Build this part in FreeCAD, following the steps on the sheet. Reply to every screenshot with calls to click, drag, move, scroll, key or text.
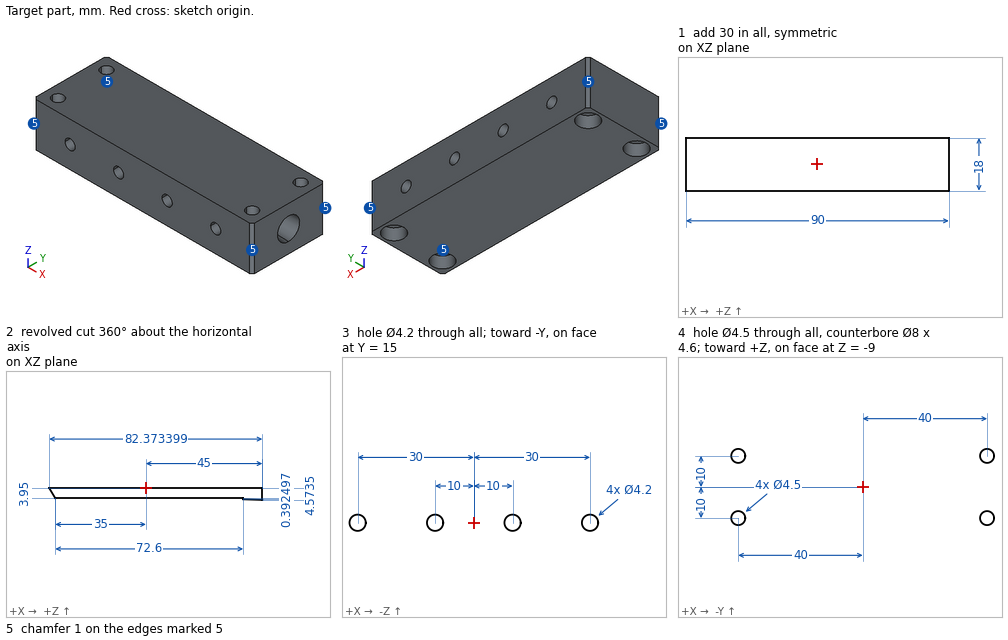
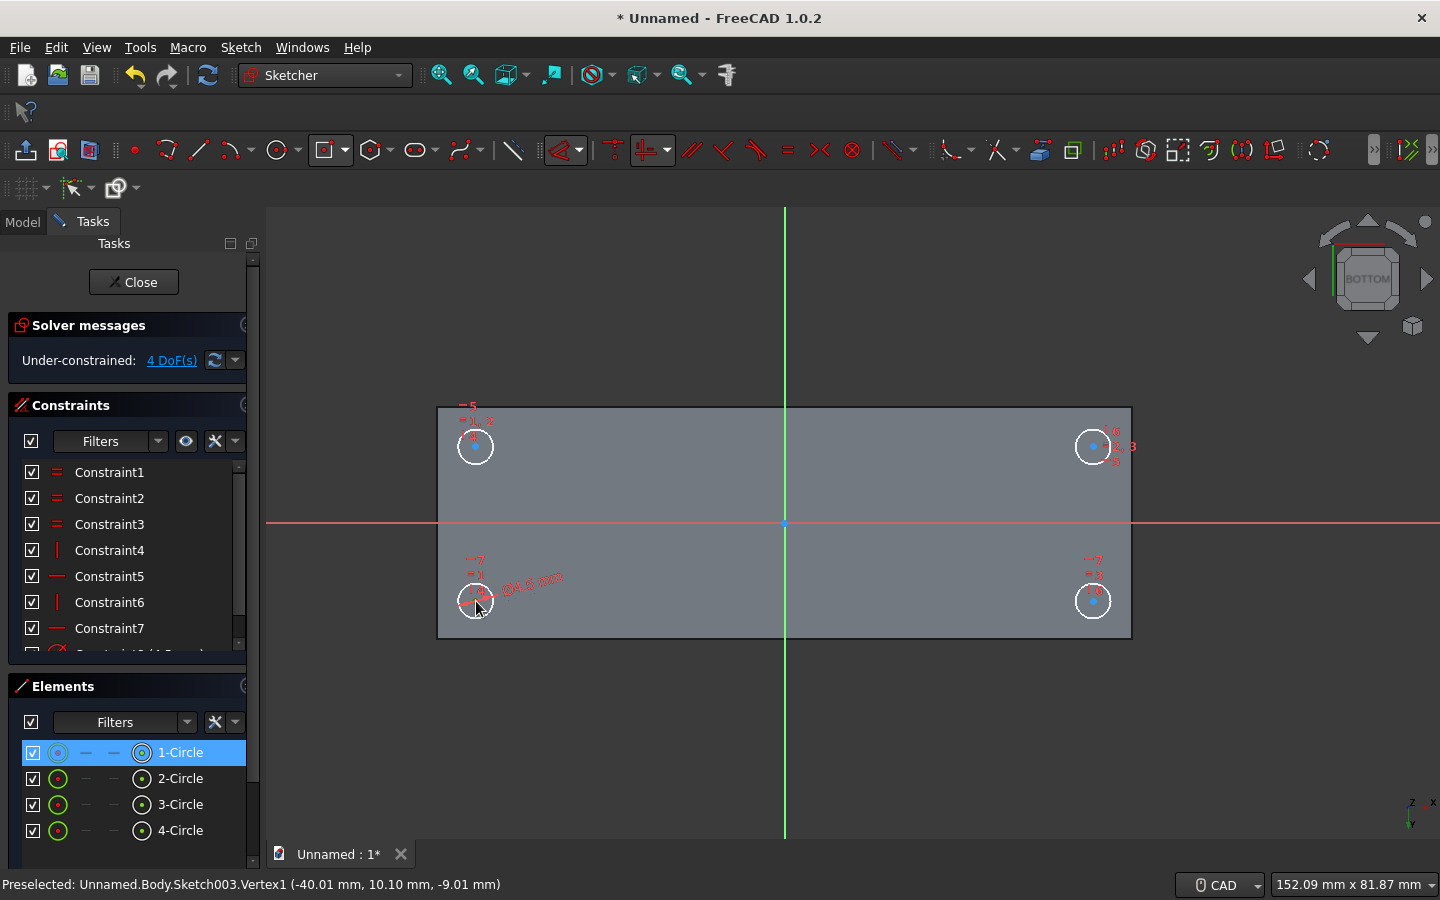
click(582, 150)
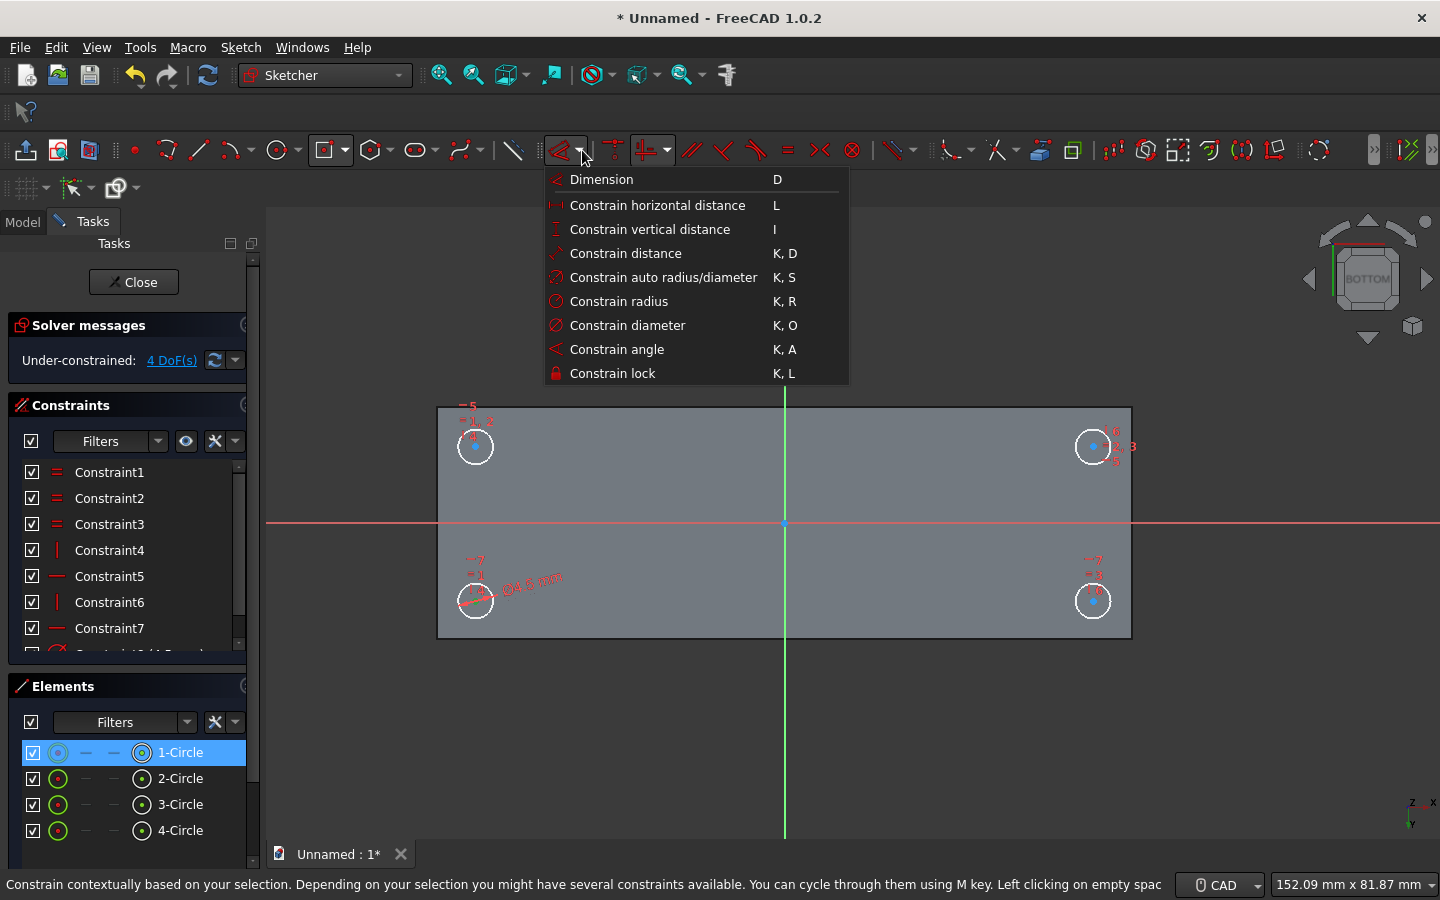
click(697, 205)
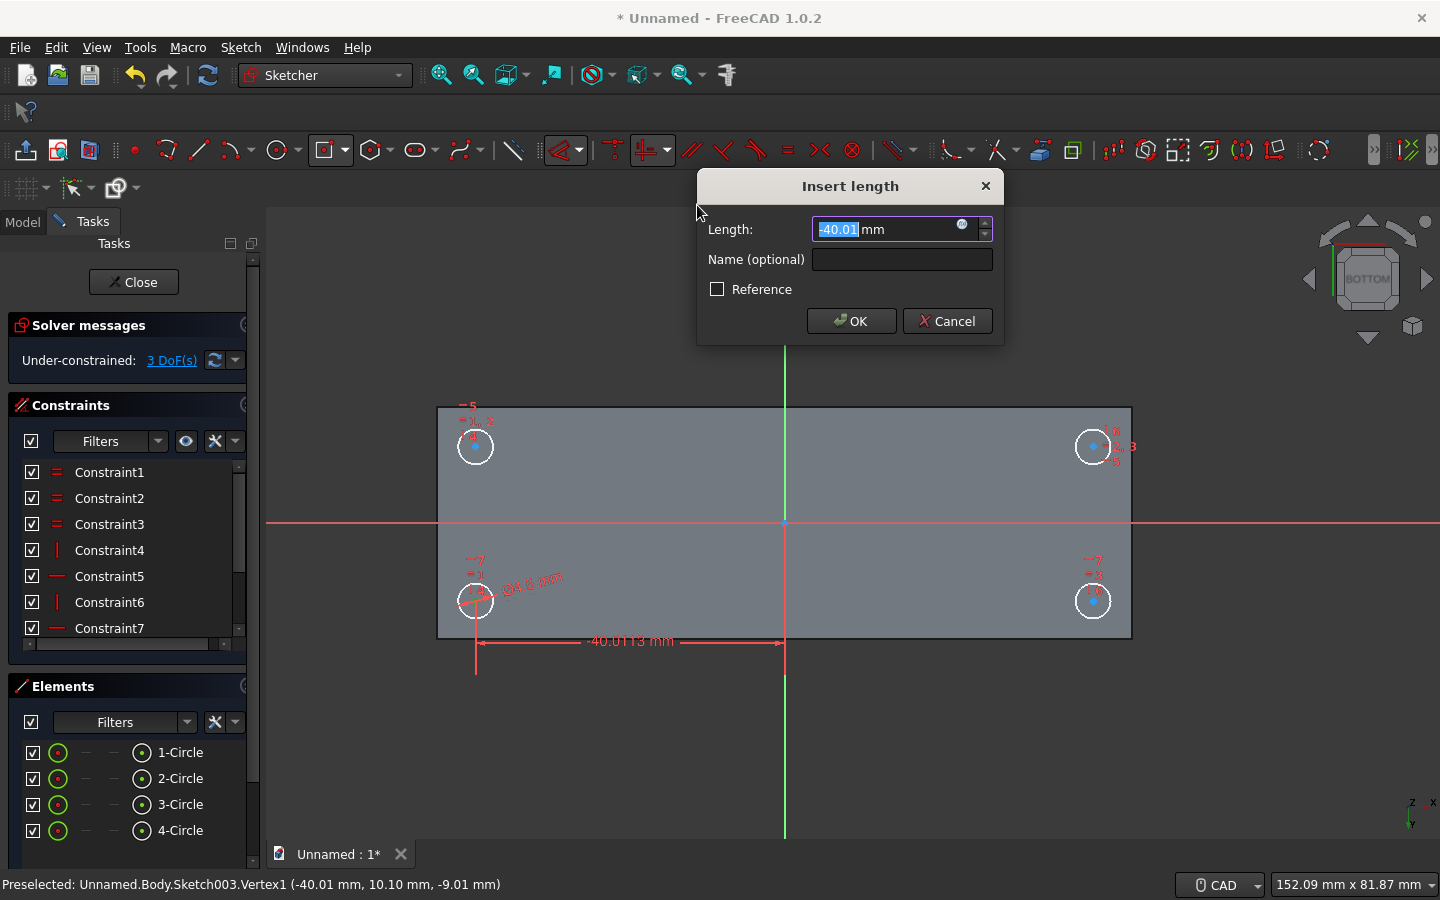
text(-40)
key(Return)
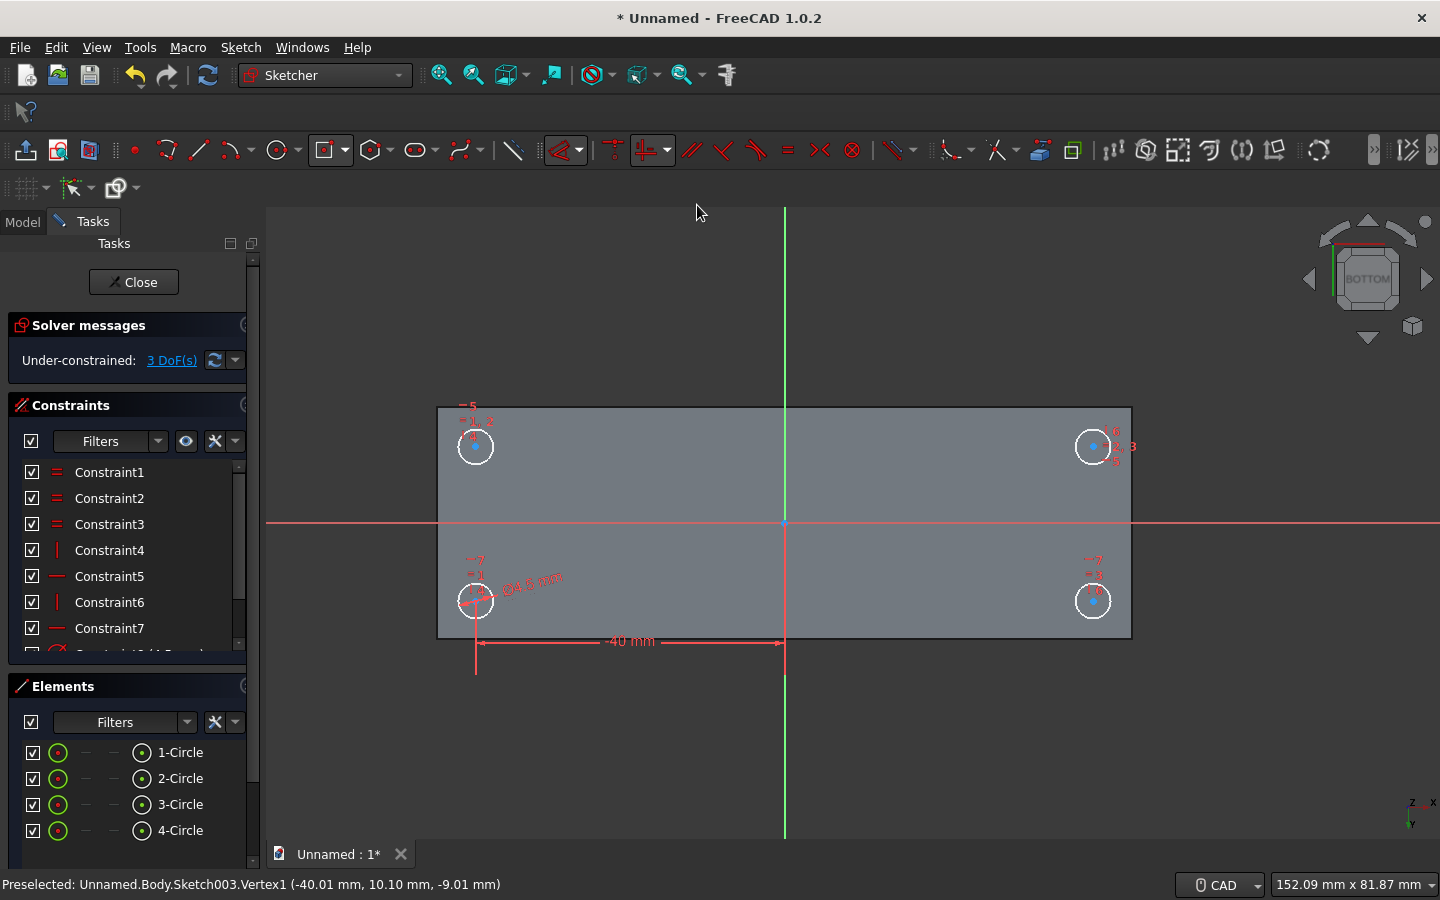
click(476, 601)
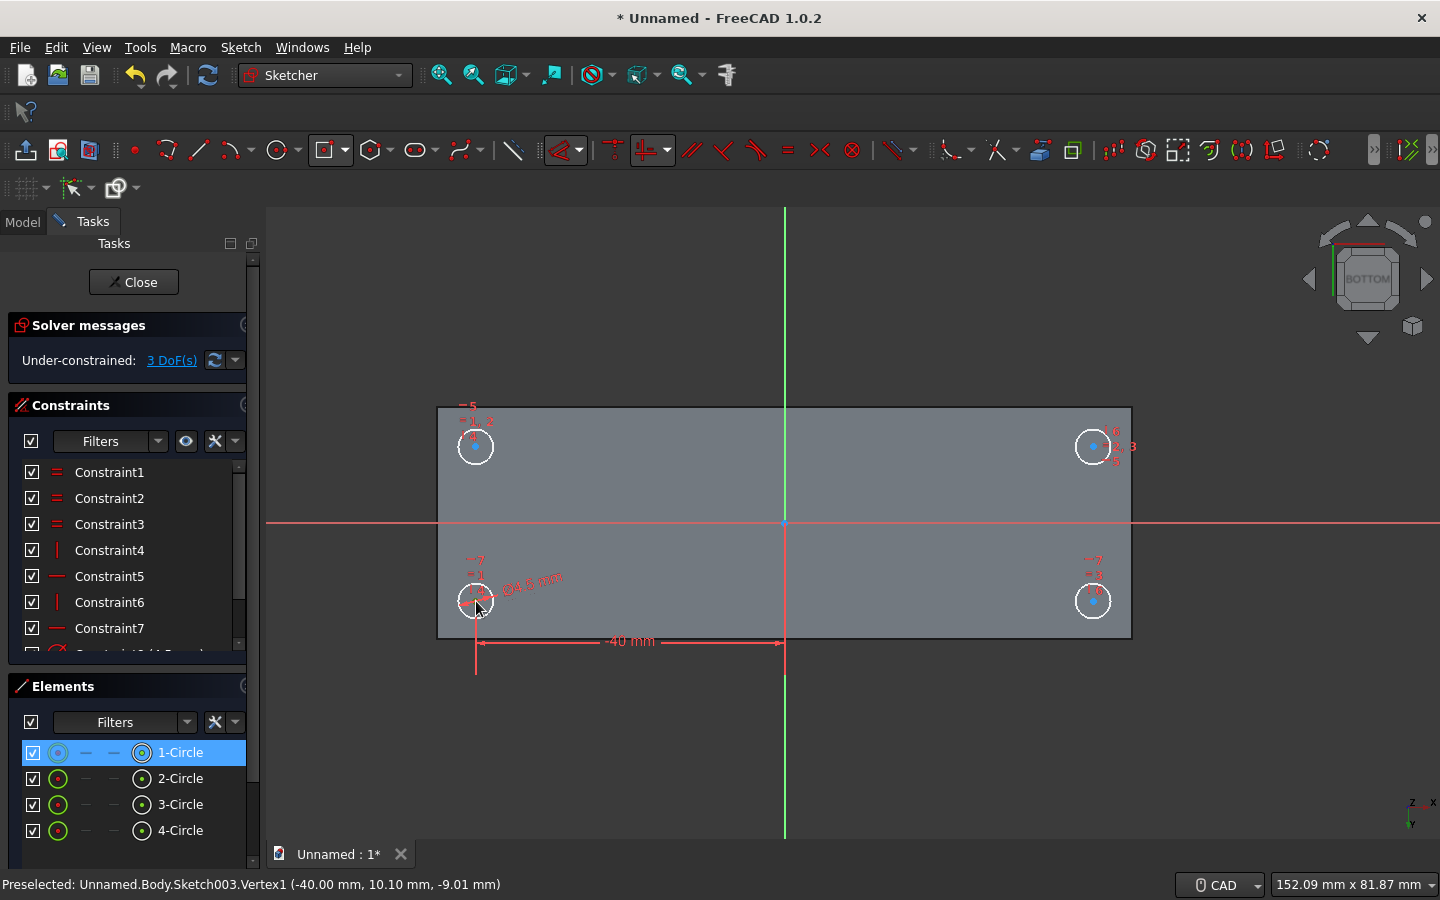
key(i)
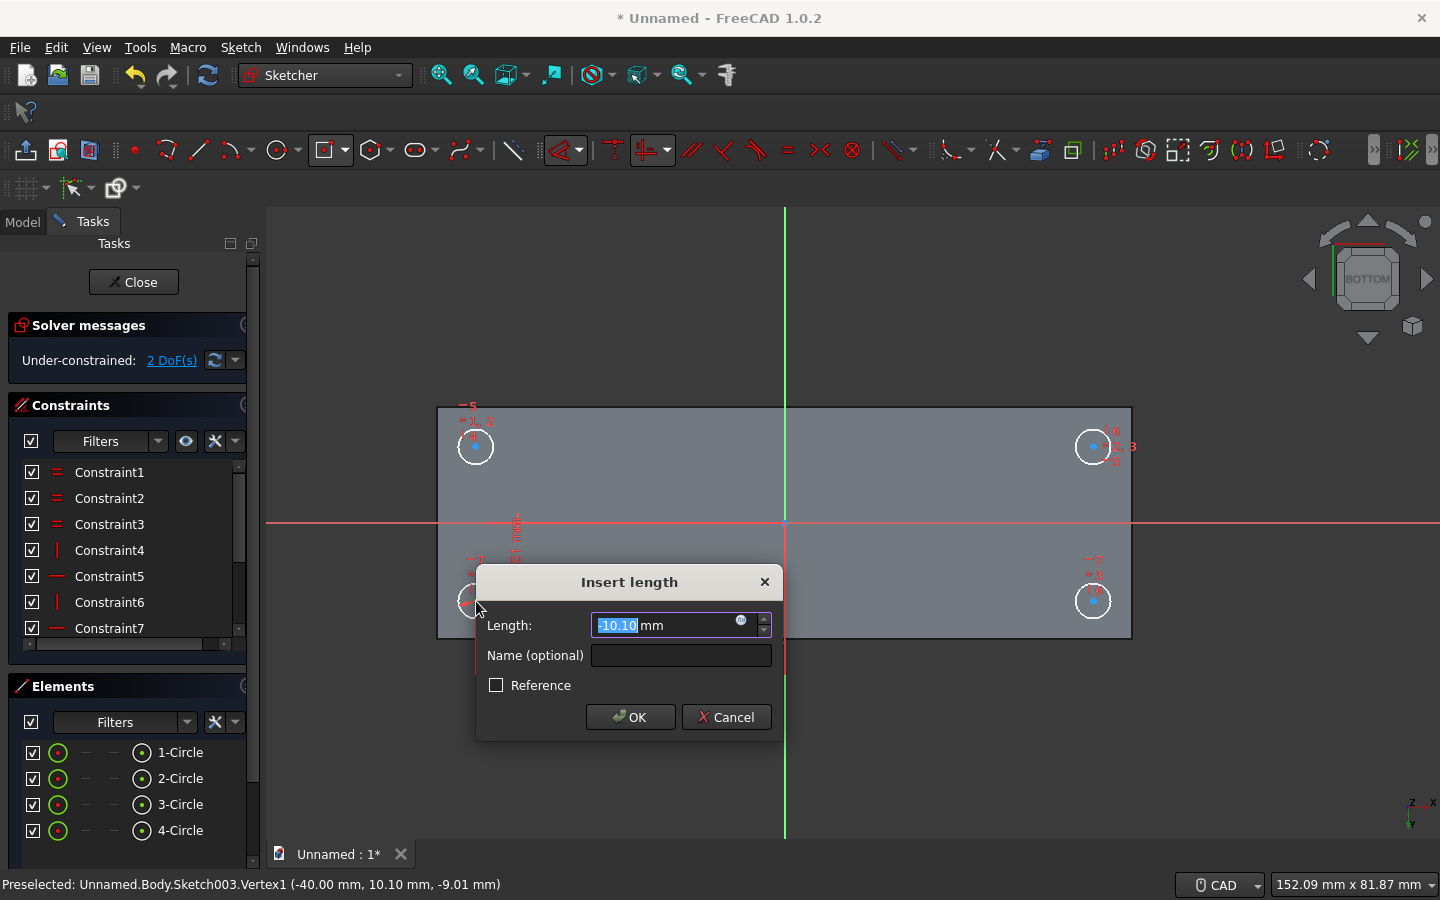
text(-10)
key(Return)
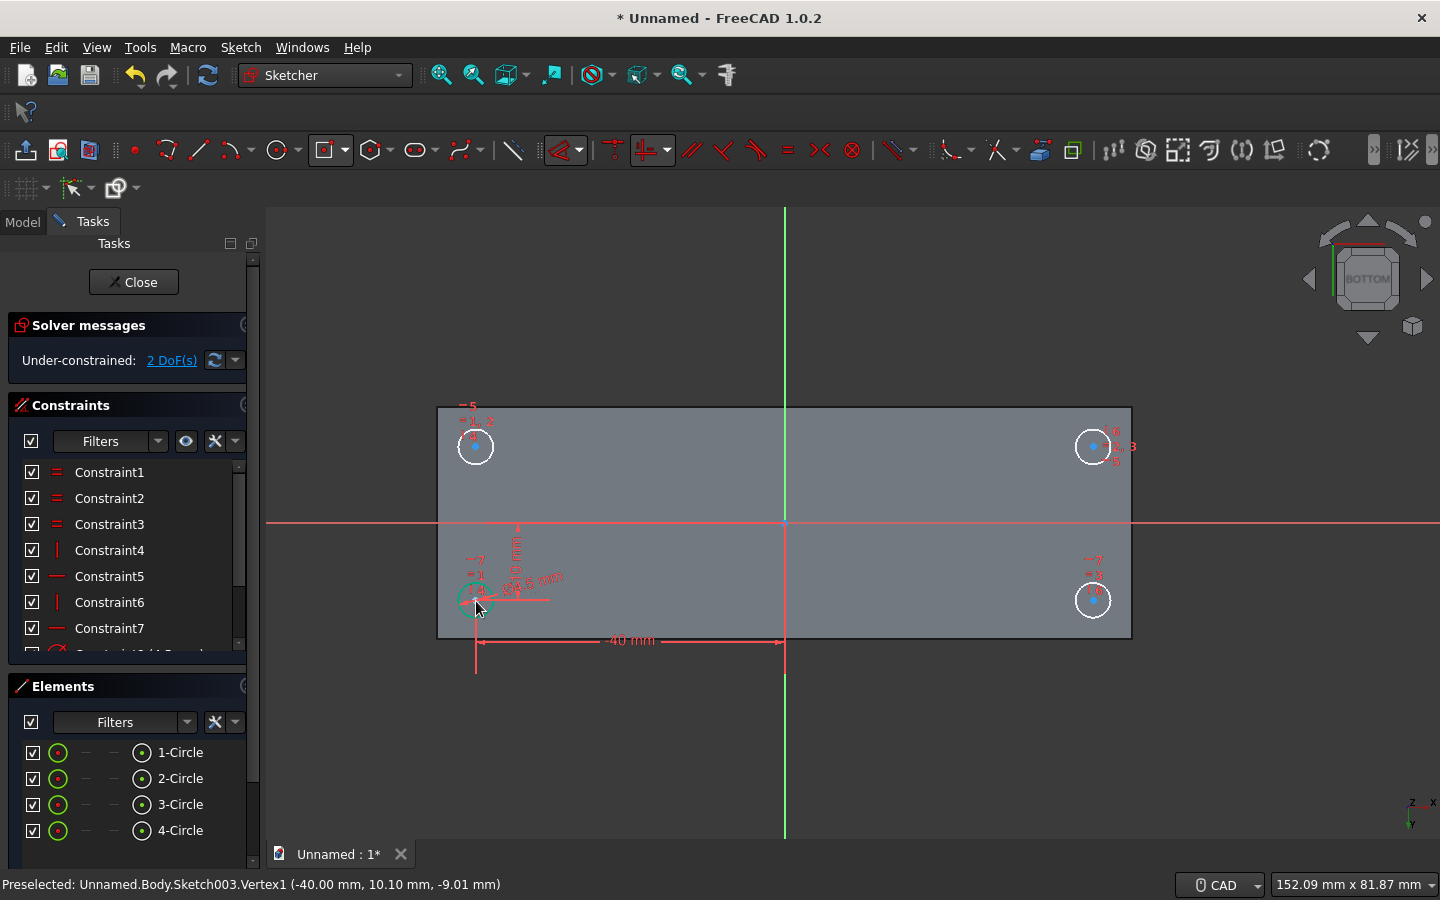
click(476, 447)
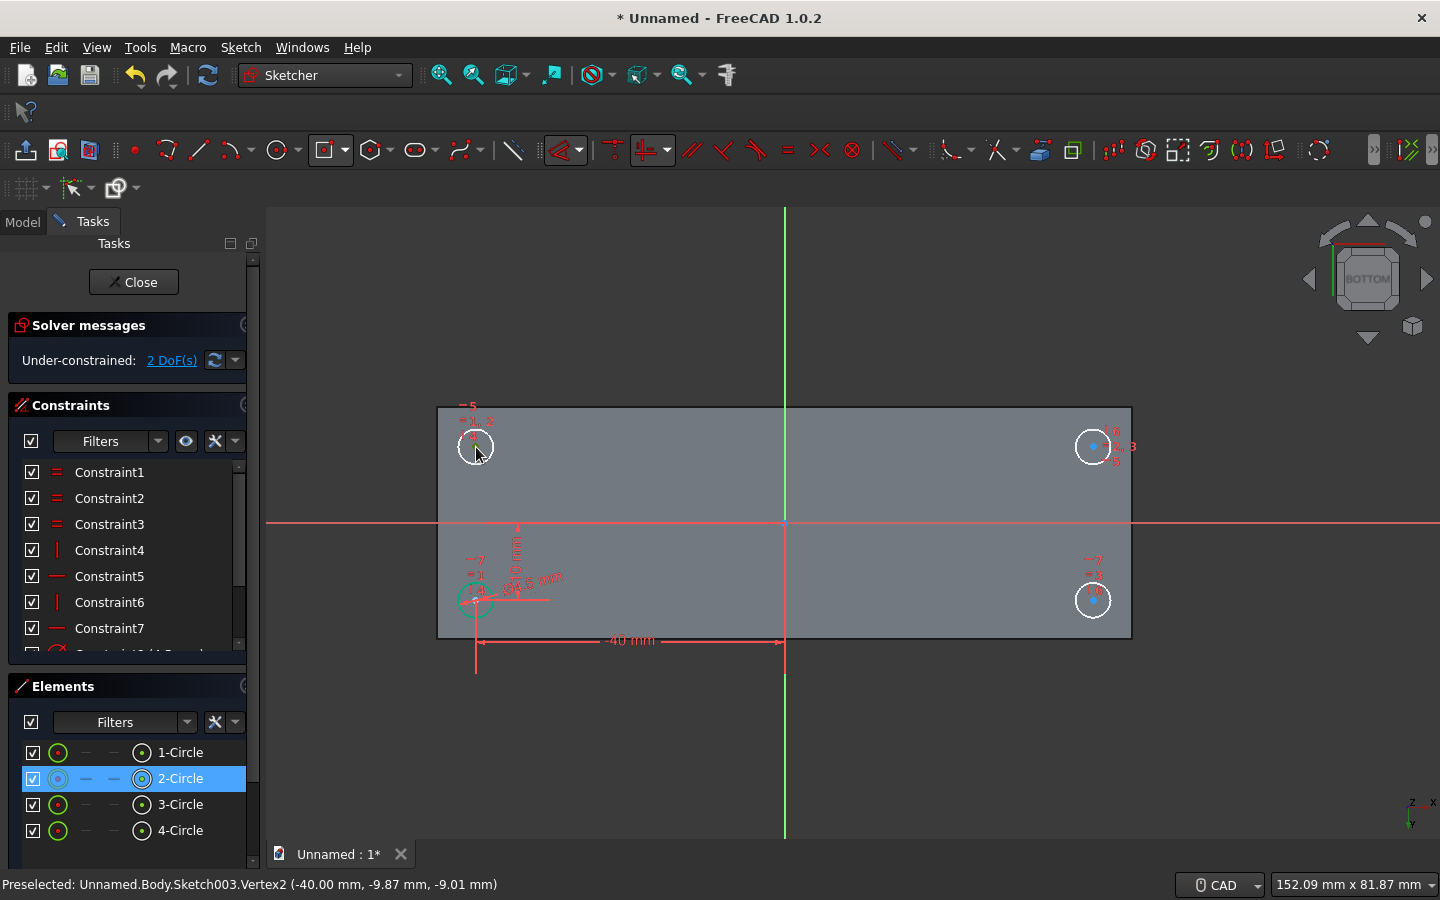
click(582, 150)